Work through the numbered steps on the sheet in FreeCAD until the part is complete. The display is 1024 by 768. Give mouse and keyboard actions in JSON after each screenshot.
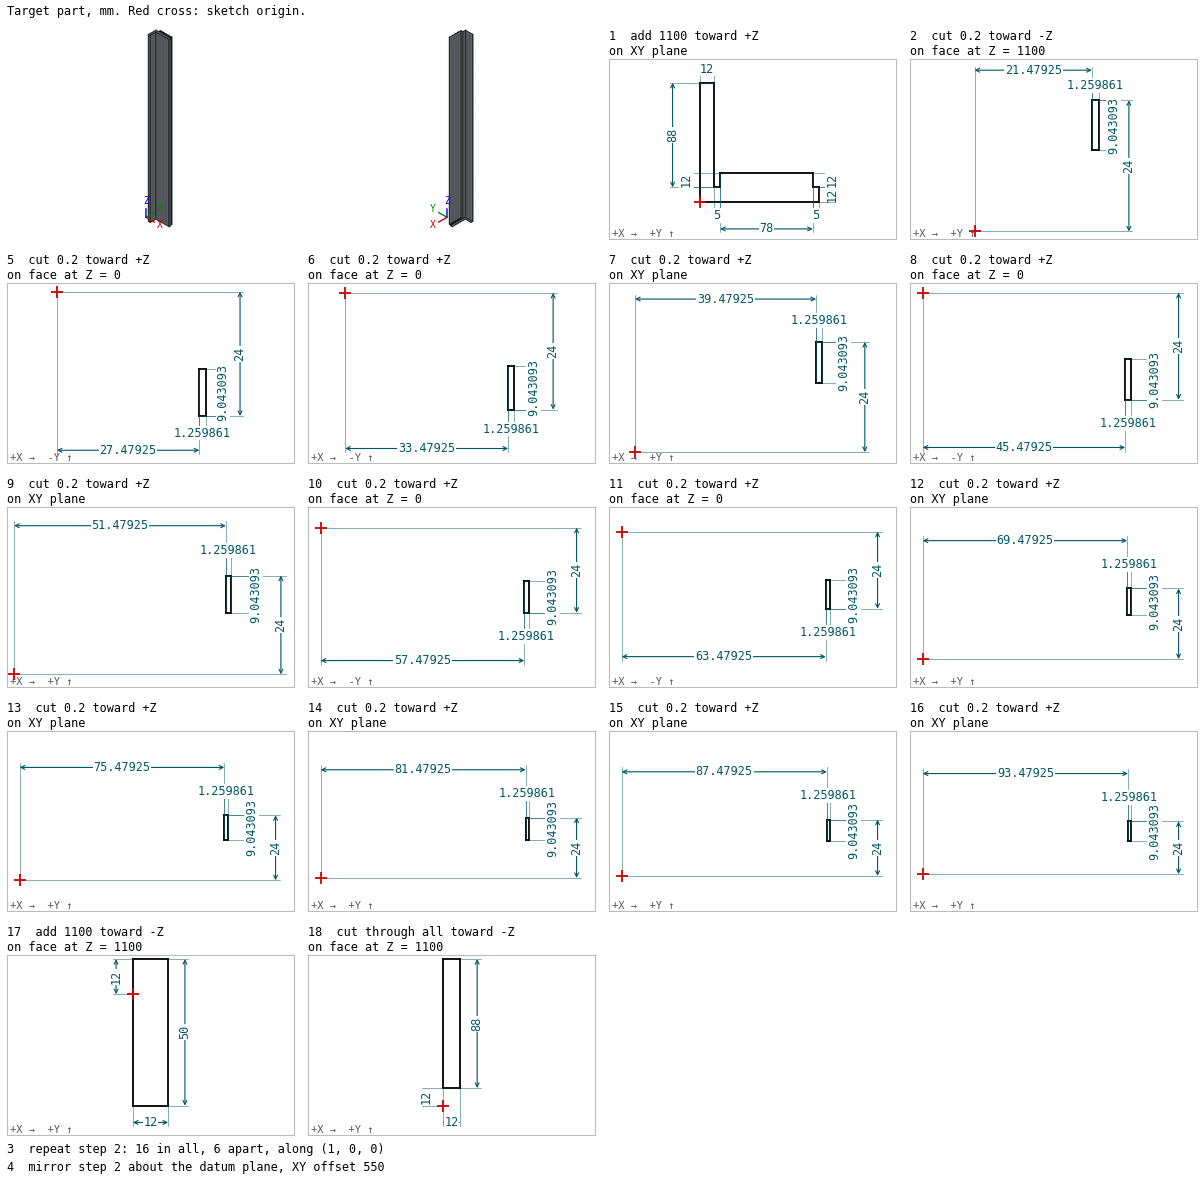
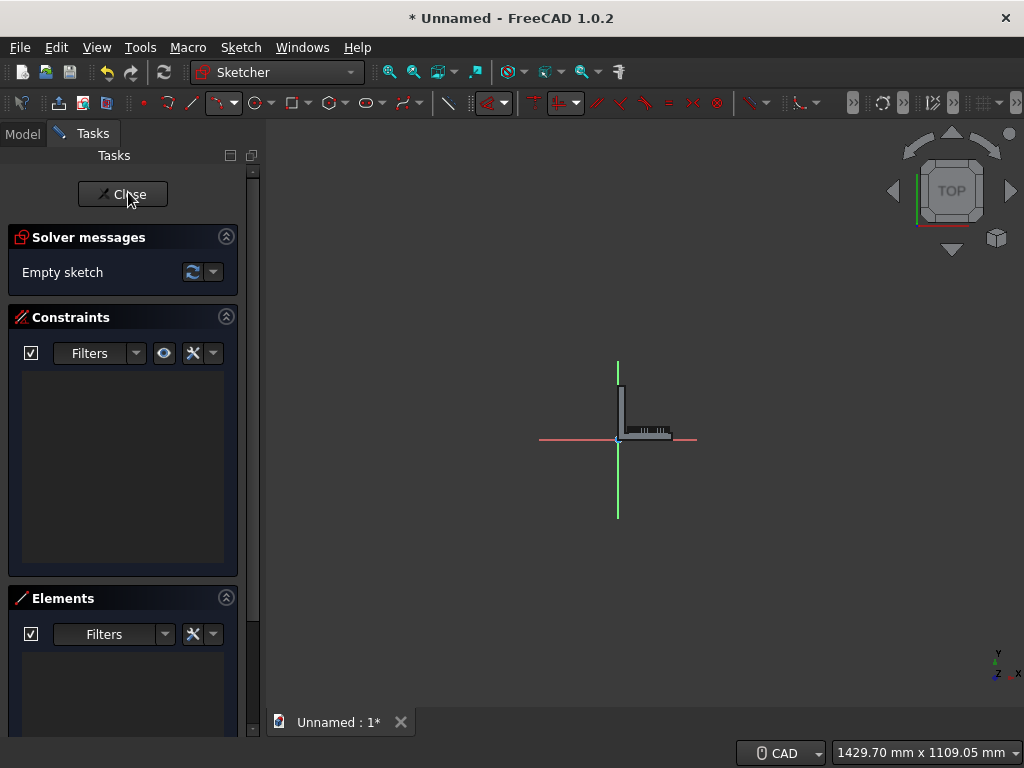
{"action": "left_click", "coordinate": [108, 104]}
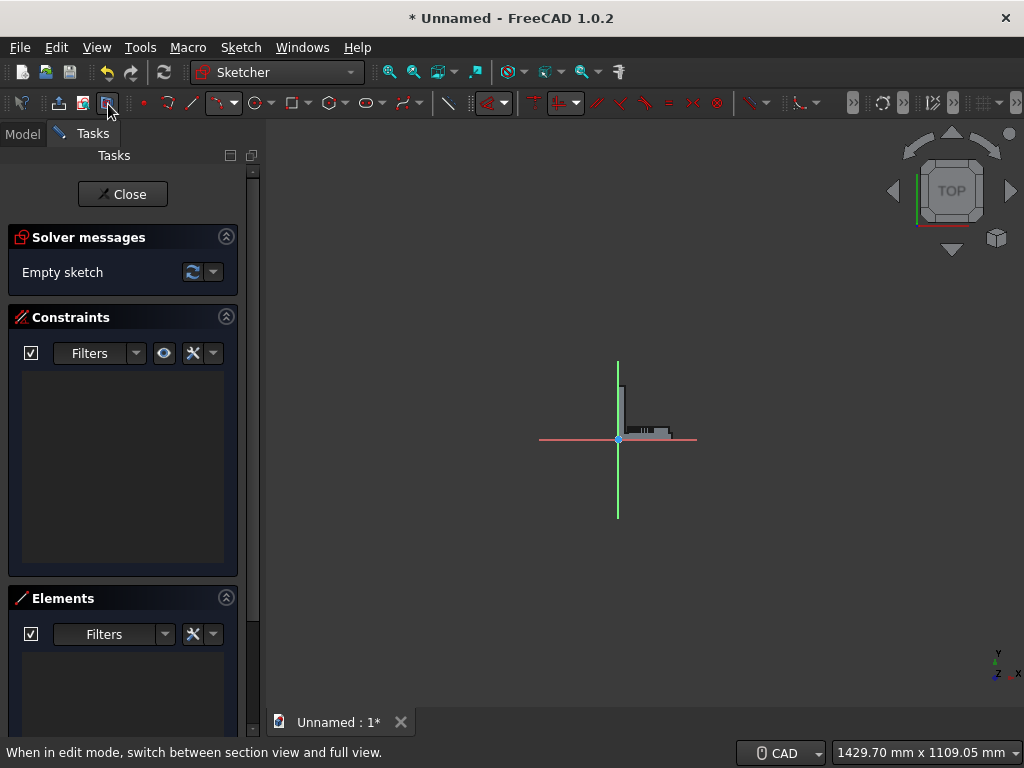
{"action": "scroll", "coordinate": [660, 430], "scroll_direction": "up", "scroll_amount": 15}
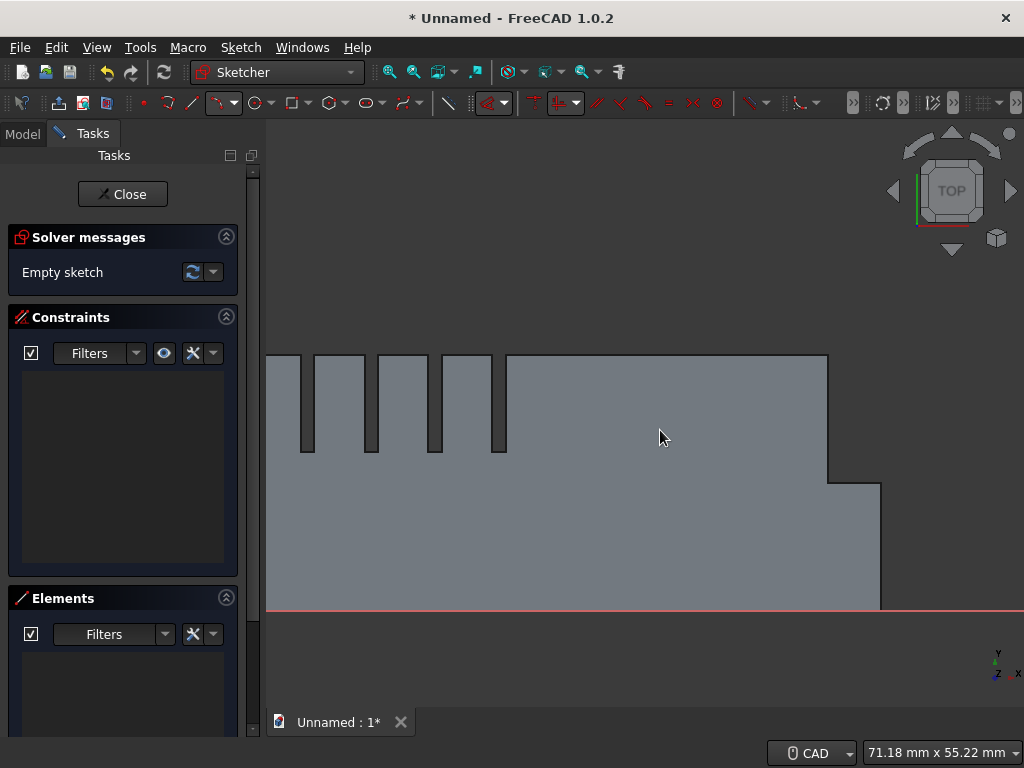
{"action": "scroll", "coordinate": [558, 400], "scroll_direction": "up", "scroll_amount": 7}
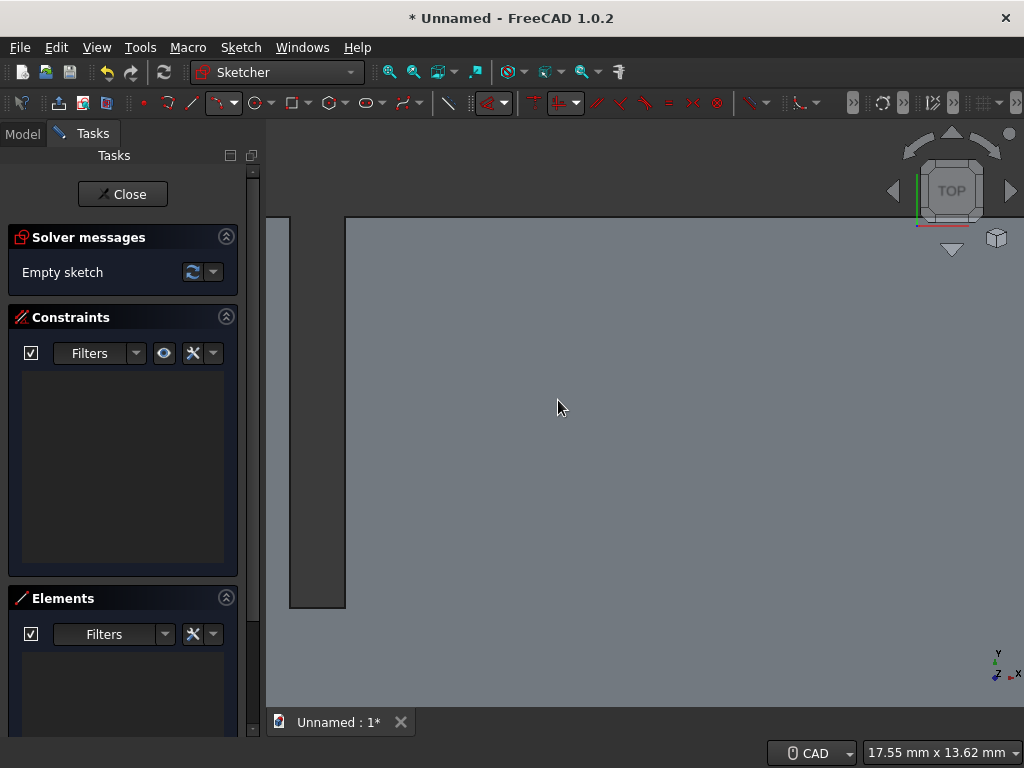
{"action": "left_click", "coordinate": [292, 104]}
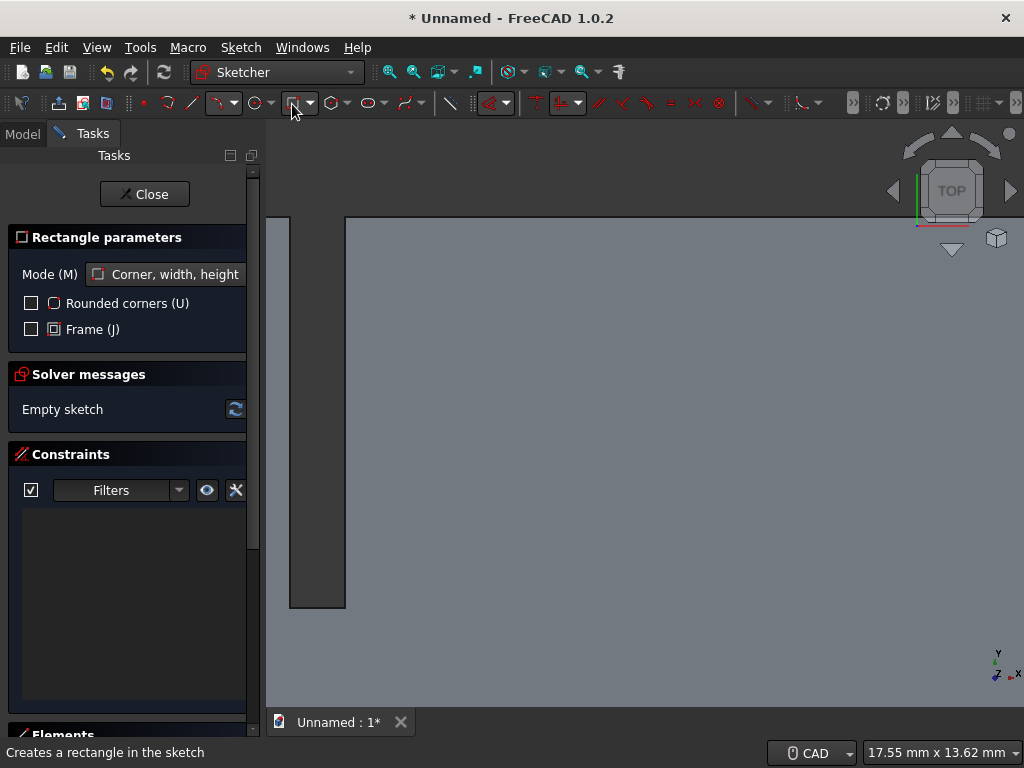
{"action": "left_click", "coordinate": [550, 217]}
{"action": "mouse_move", "coordinate": [604, 608]}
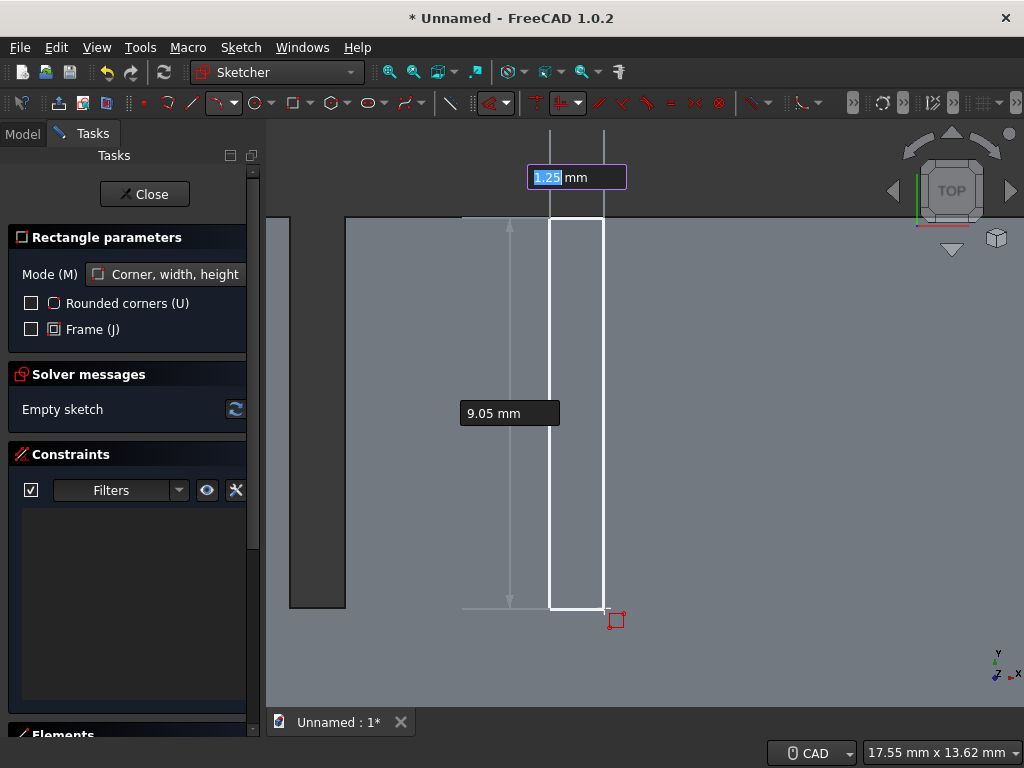
{"action": "type", "text": "1.259861"}
{"action": "key", "text": "Tab"}
{"action": "type", "text": "9.043093"}
{"action": "key", "text": "Return"}
{"action": "key", "text": "Escape"}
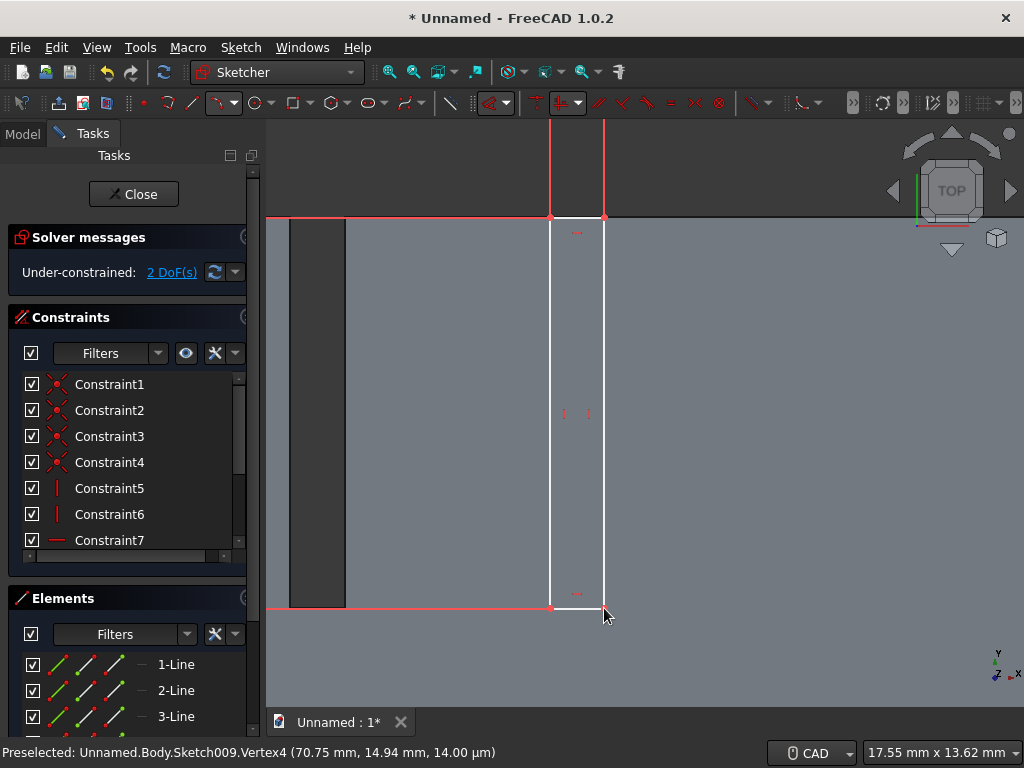
{"action": "left_click", "coordinate": [550, 218]}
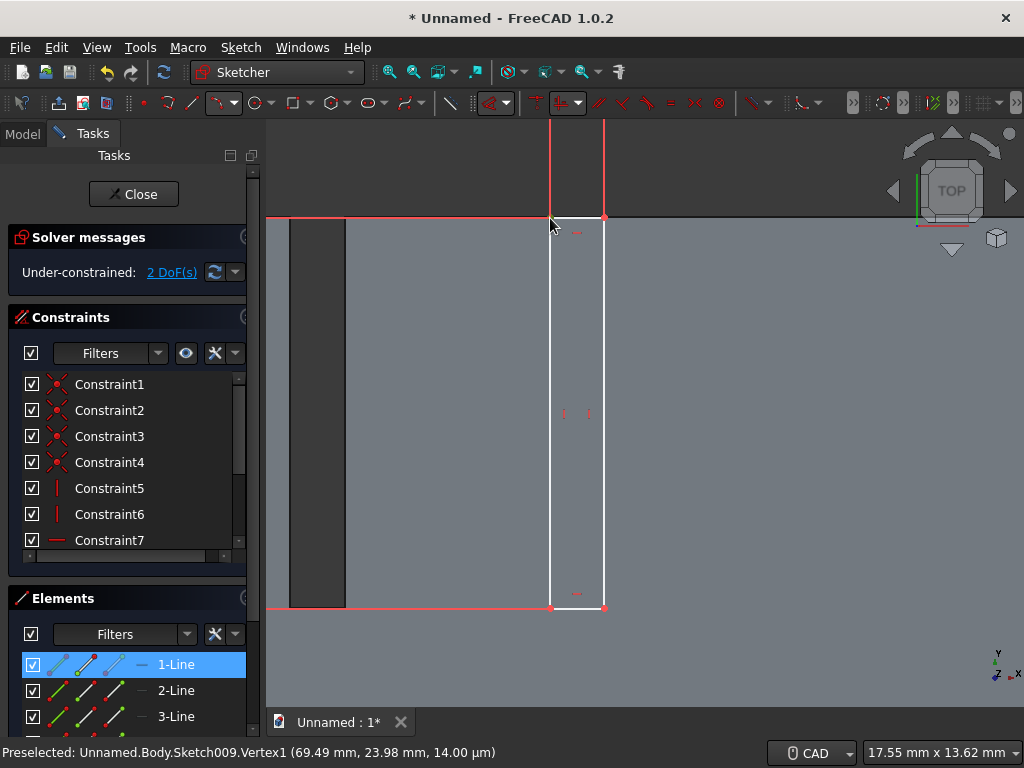
{"action": "left_click", "coordinate": [508, 104]}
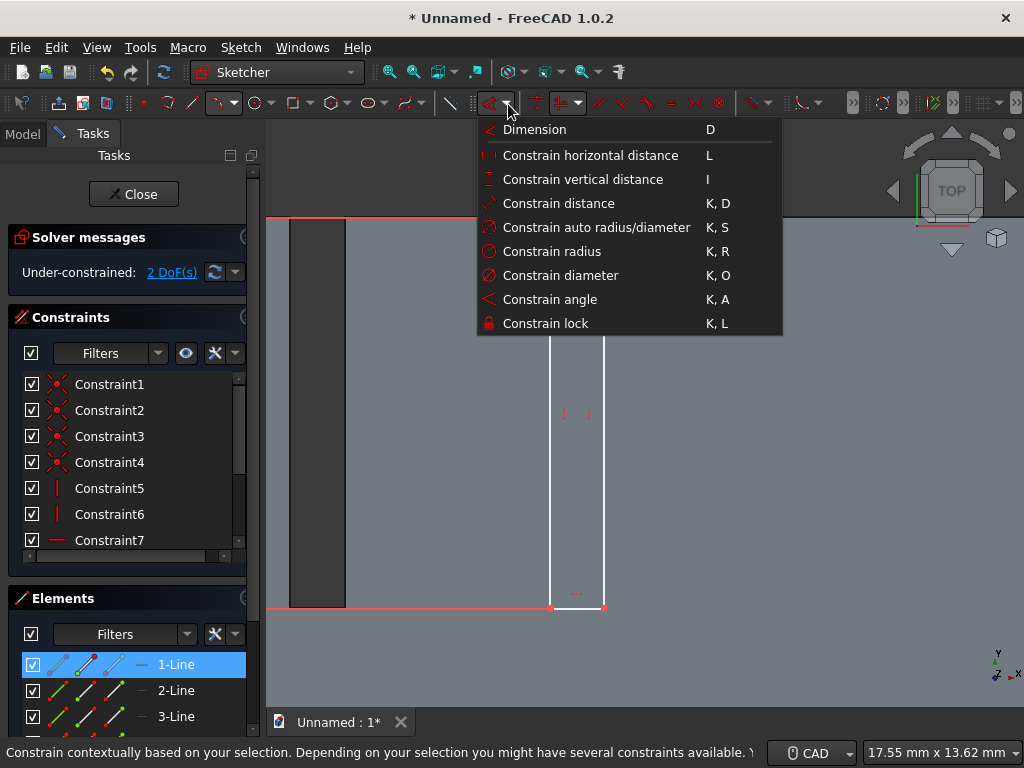
{"action": "left_click", "coordinate": [630, 179]}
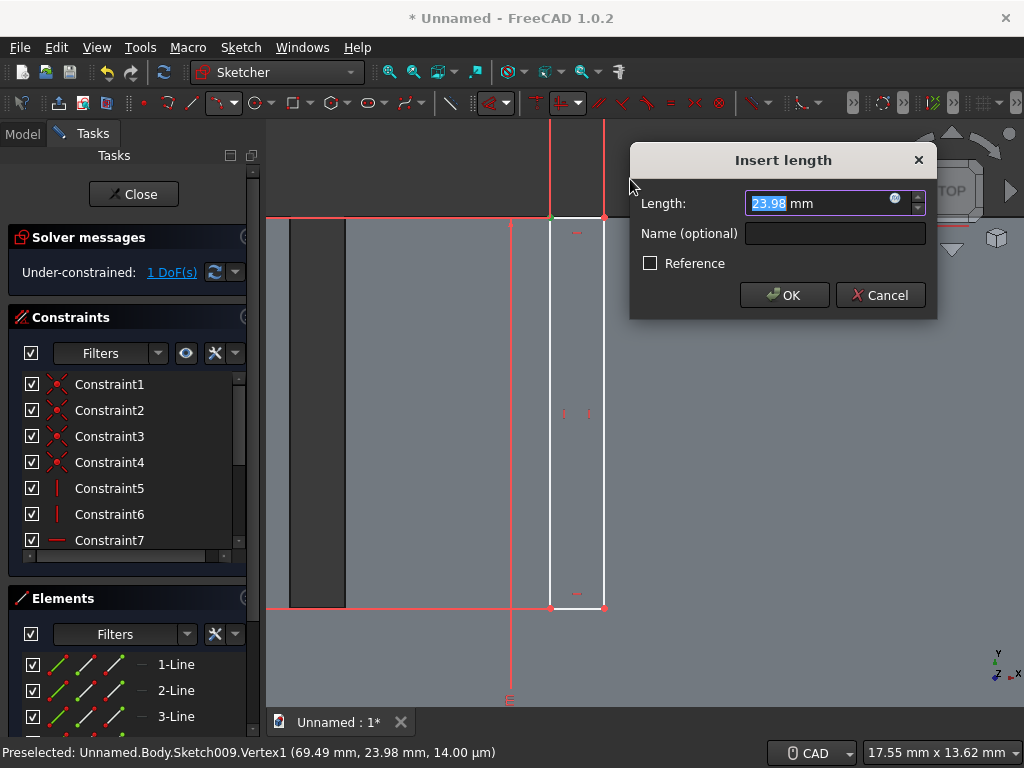
{"action": "type", "text": "24"}
{"action": "key", "text": "Return"}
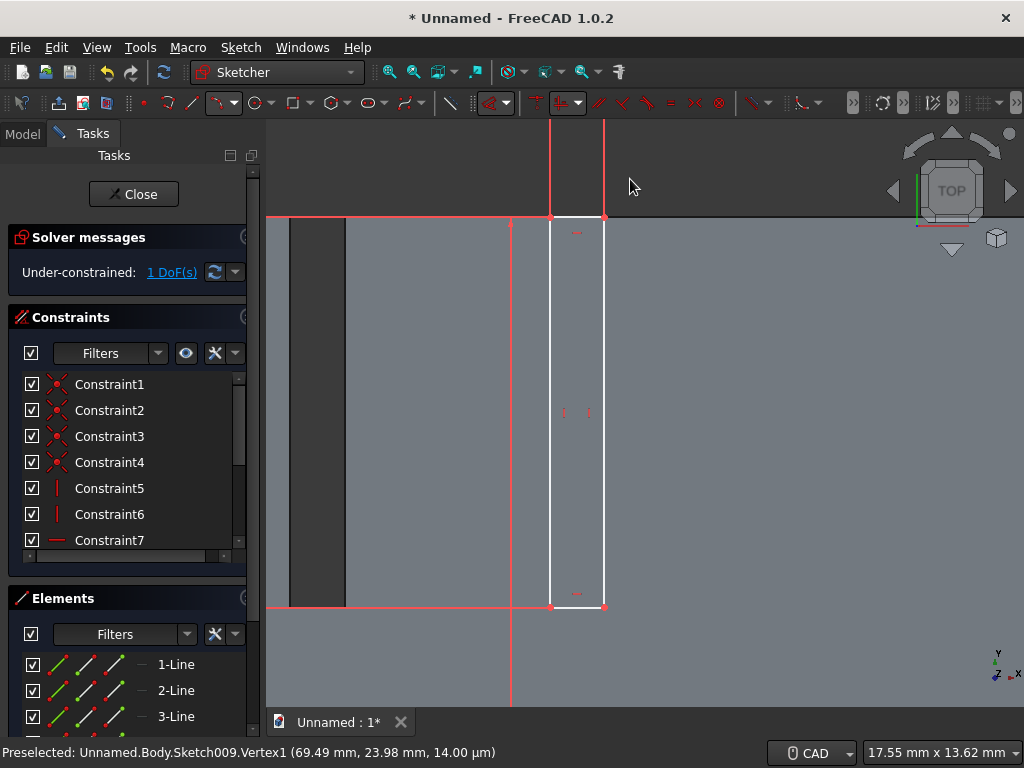
{"action": "left_click", "coordinate": [550, 217]}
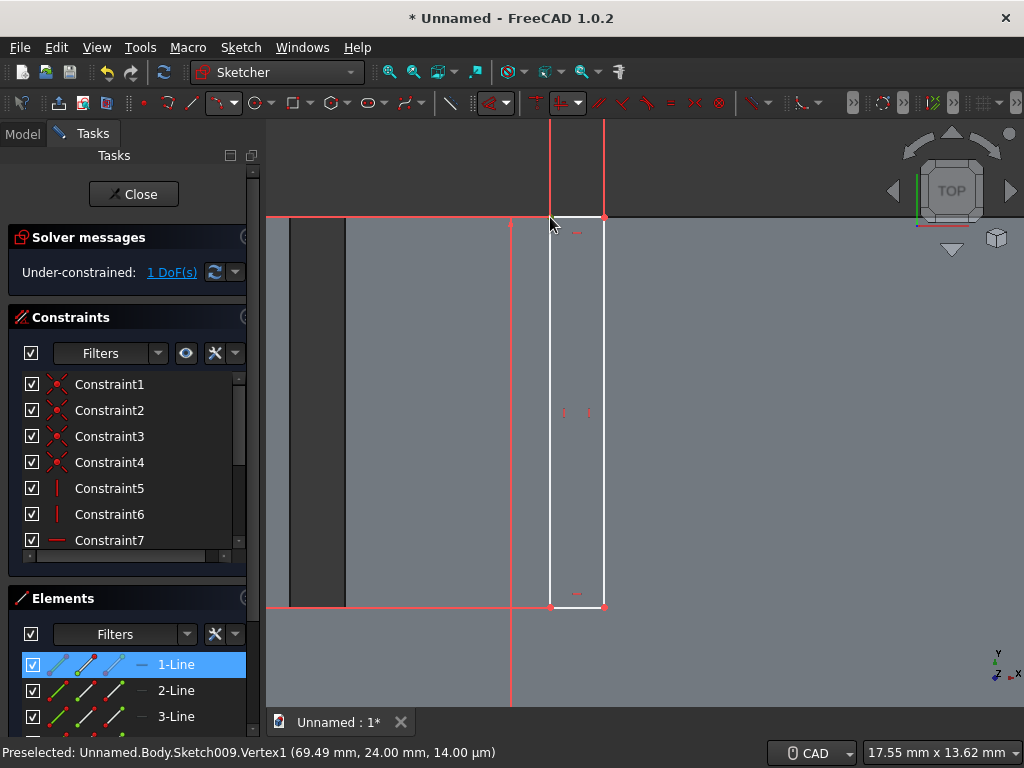
{"action": "key", "text": "l"}